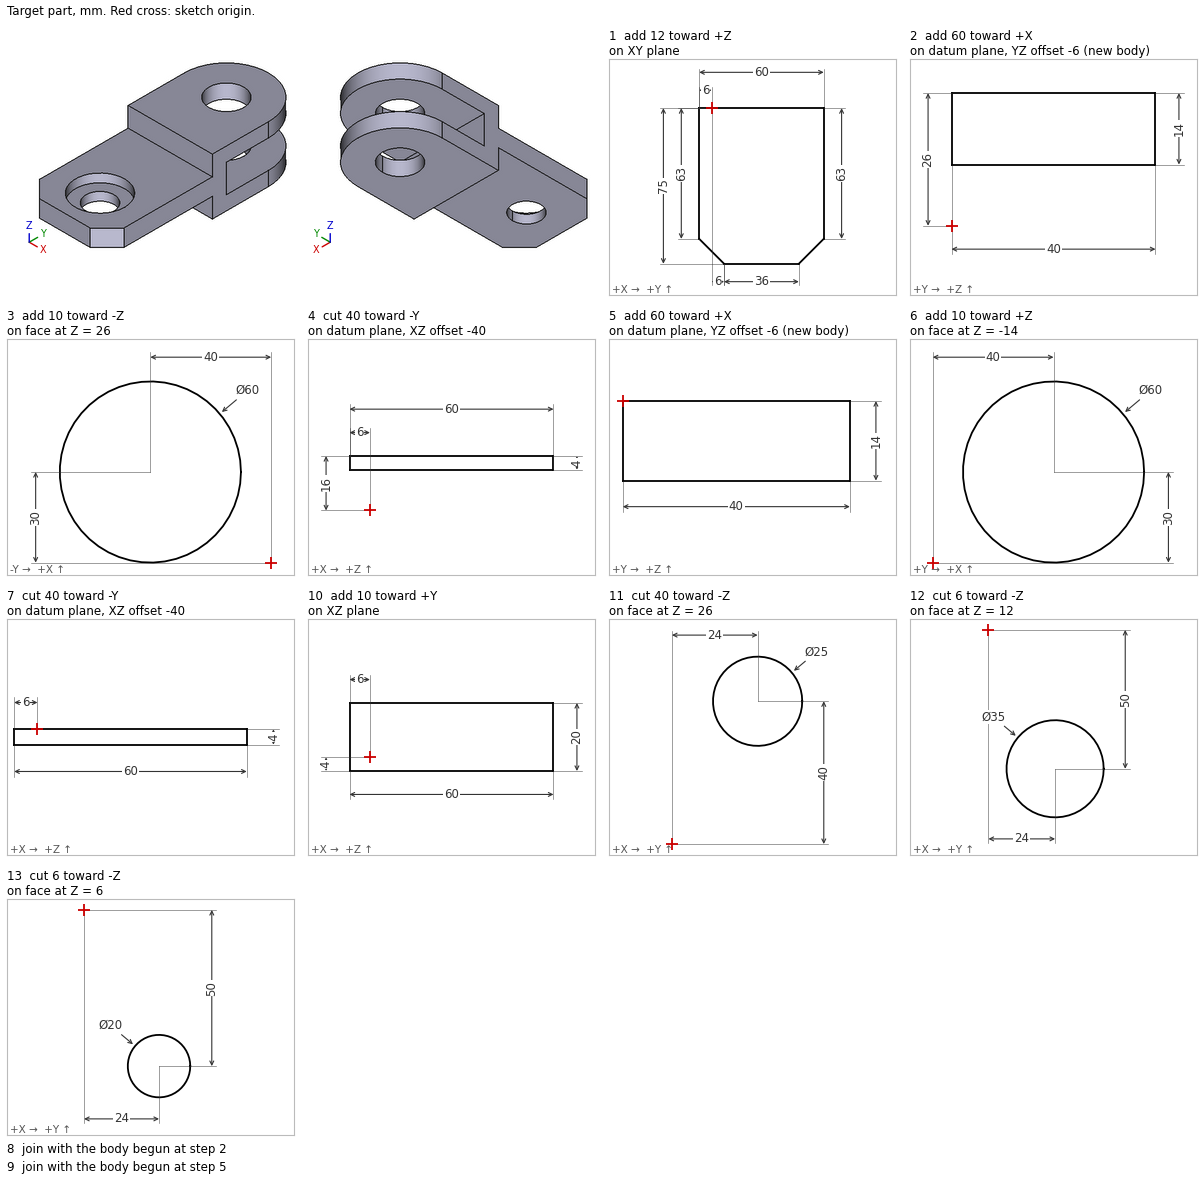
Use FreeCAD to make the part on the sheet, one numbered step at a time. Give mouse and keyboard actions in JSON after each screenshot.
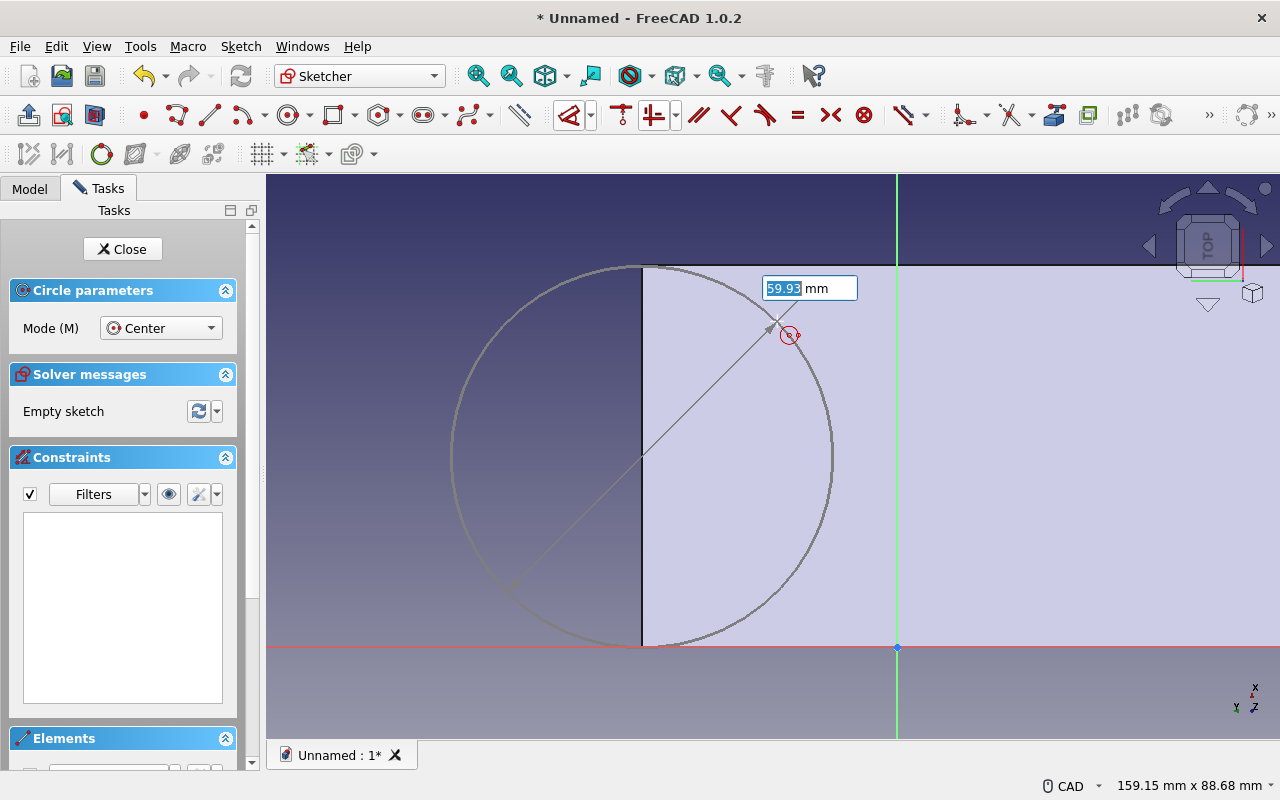
{"action": "type", "text": "60"}
{"action": "key", "text": "Return"}
{"action": "key", "text": "Escape"}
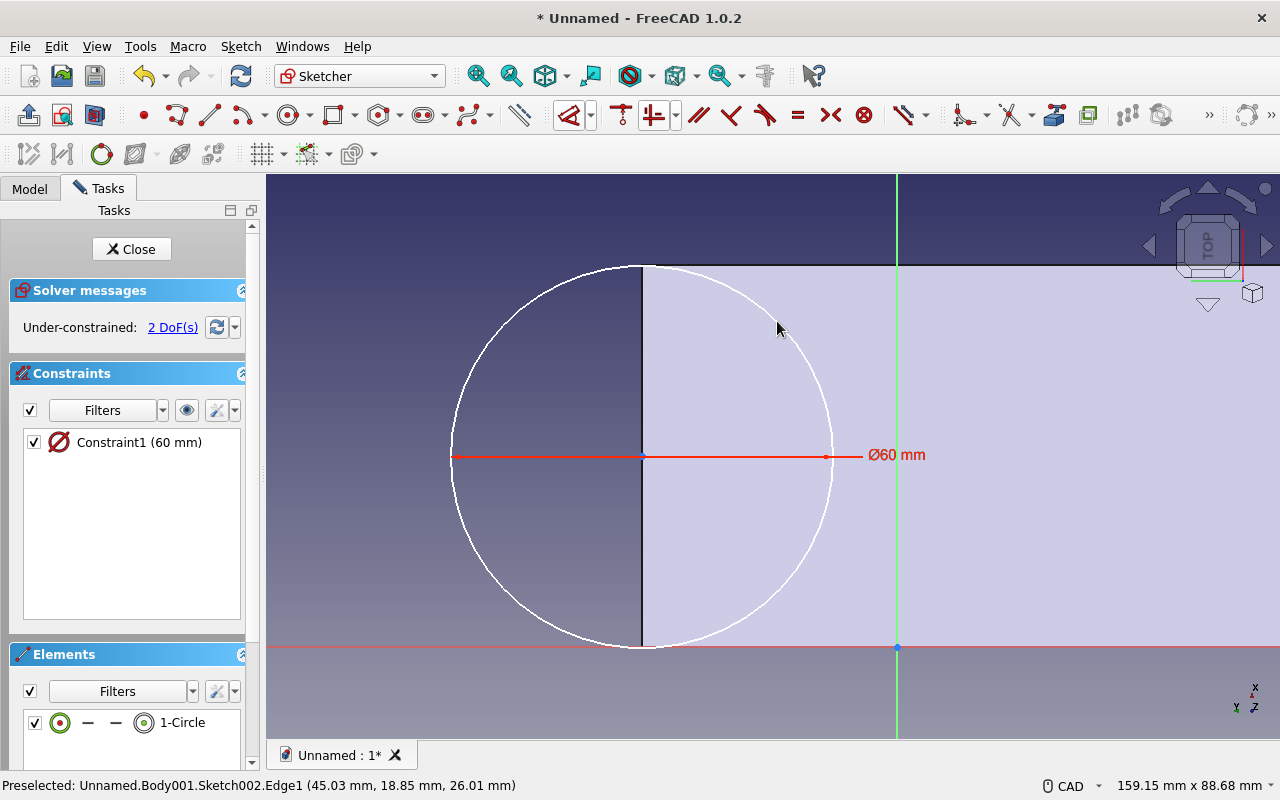
{"action": "left_click", "coordinate": [642, 457]}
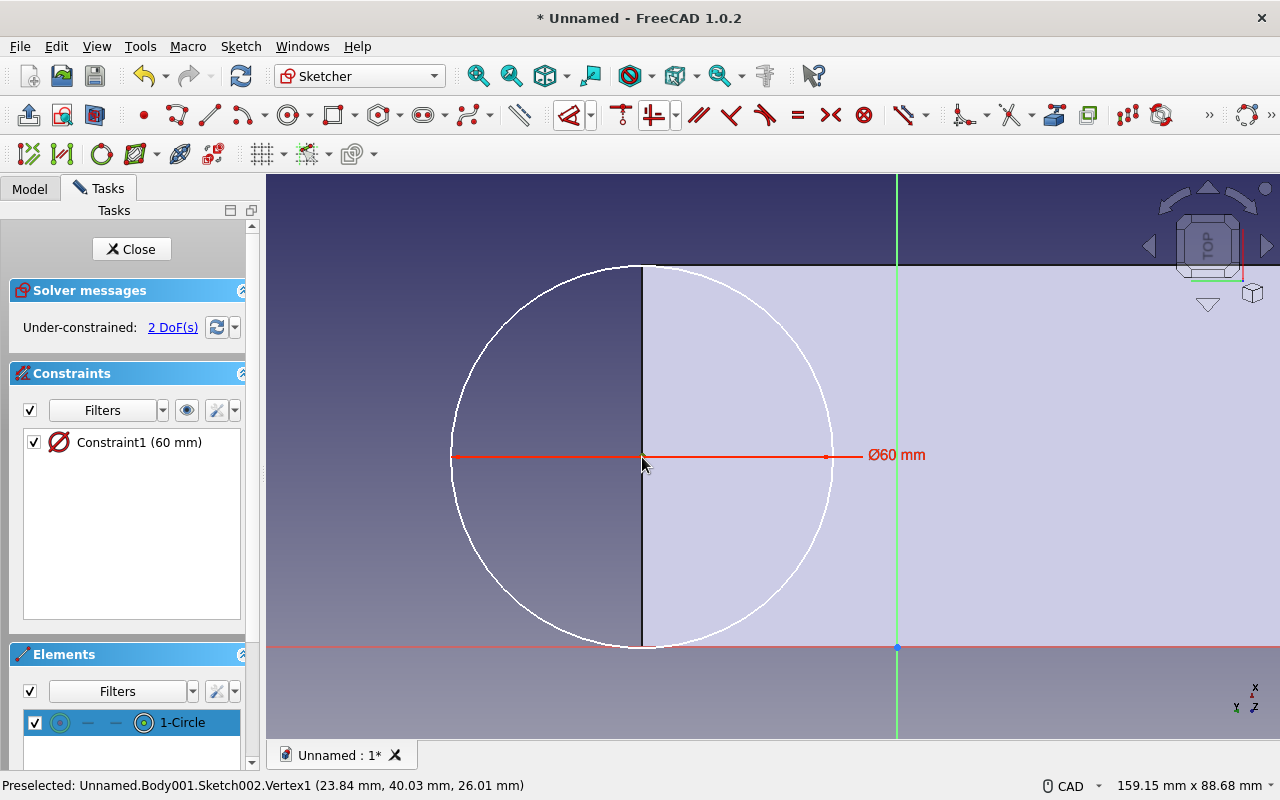
{"action": "left_click", "coordinate": [590, 116]}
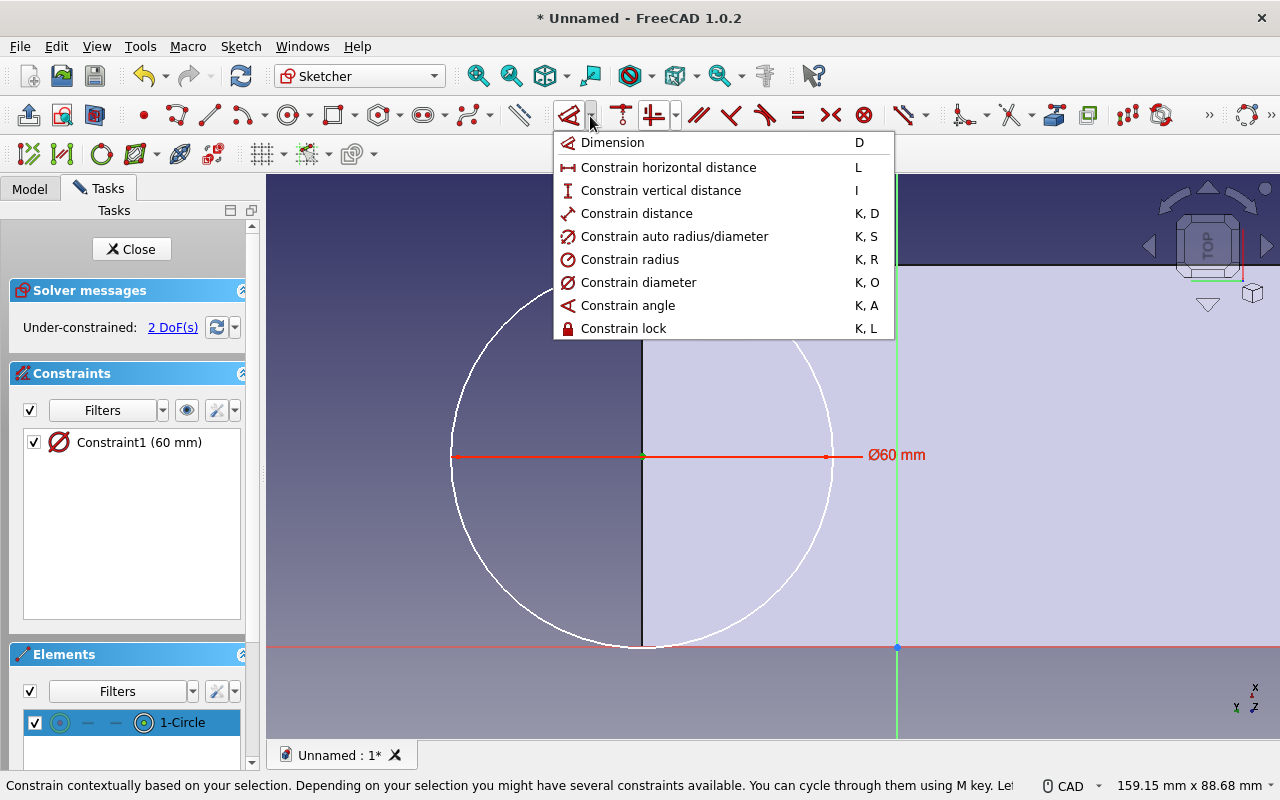
{"action": "left_click", "coordinate": [724, 168]}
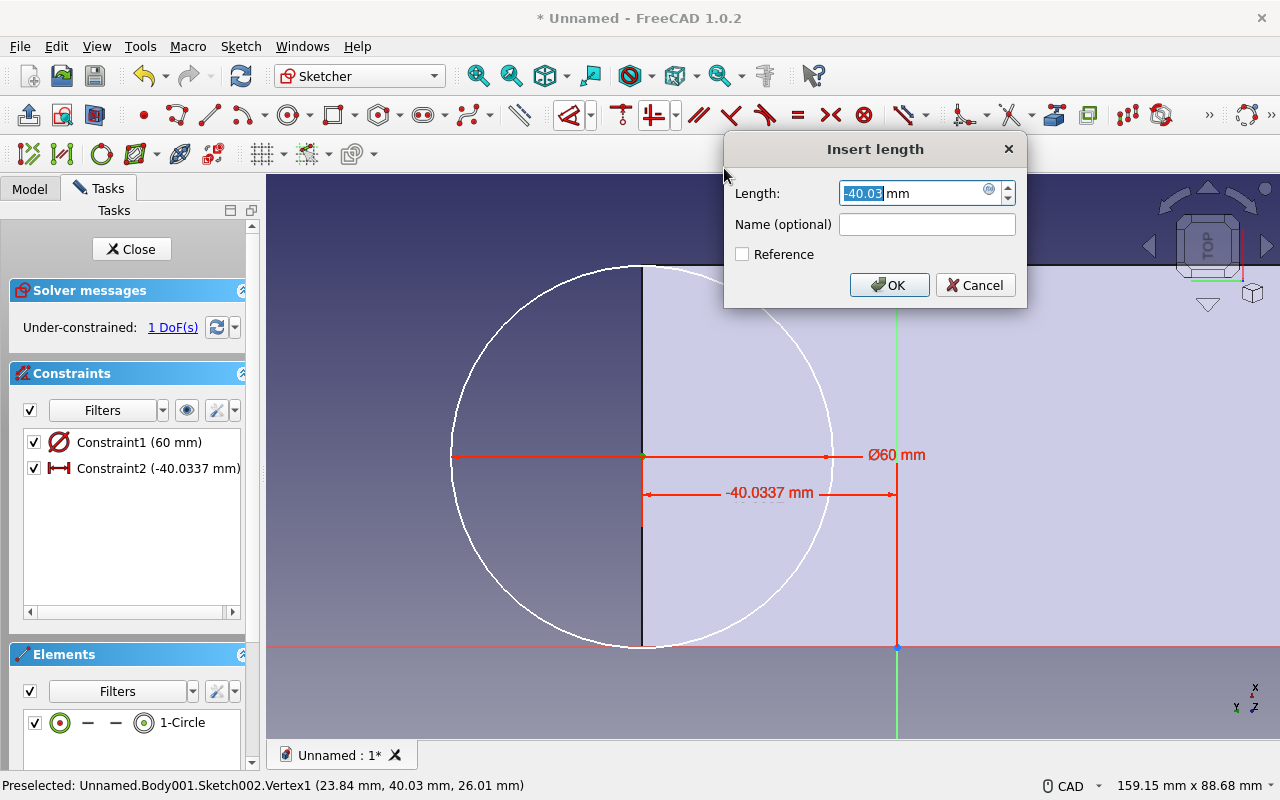
{"action": "type", "text": "-40"}
{"action": "key", "text": "Return"}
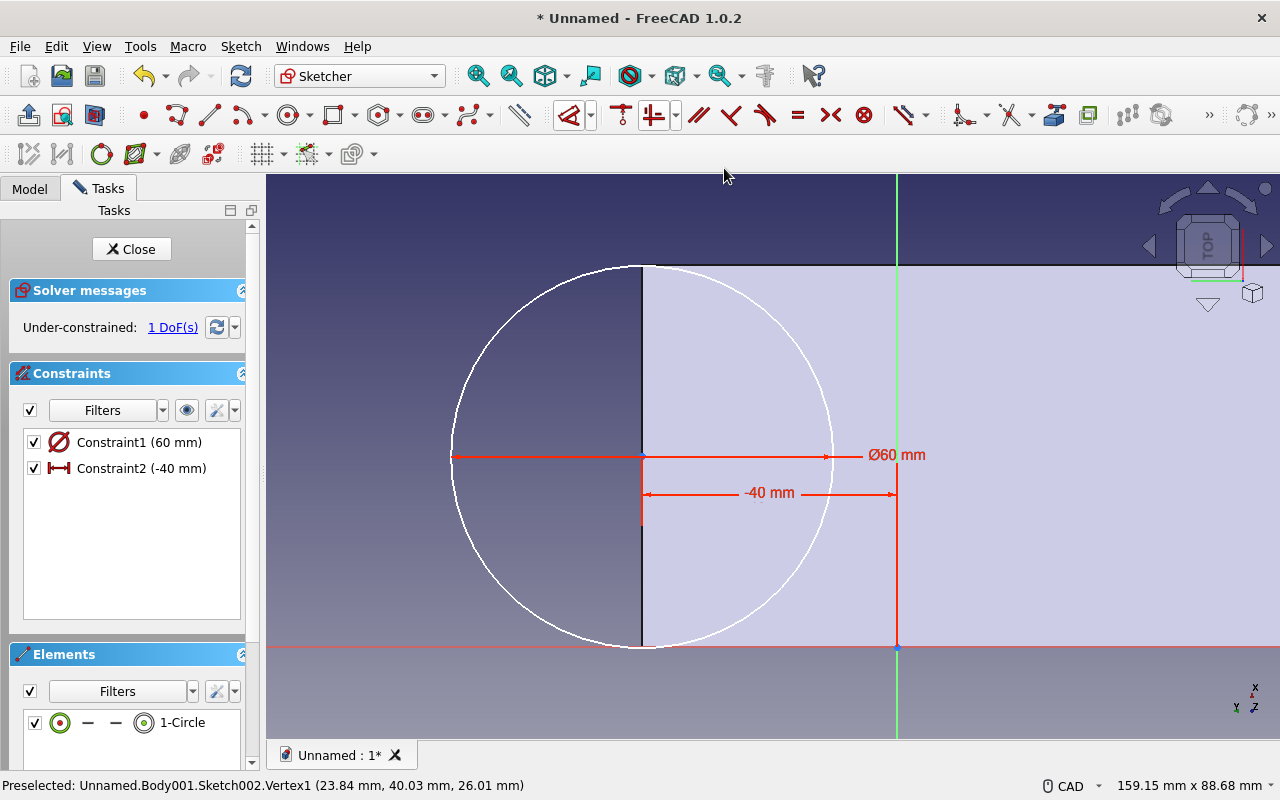
{"action": "left_click", "coordinate": [642, 457]}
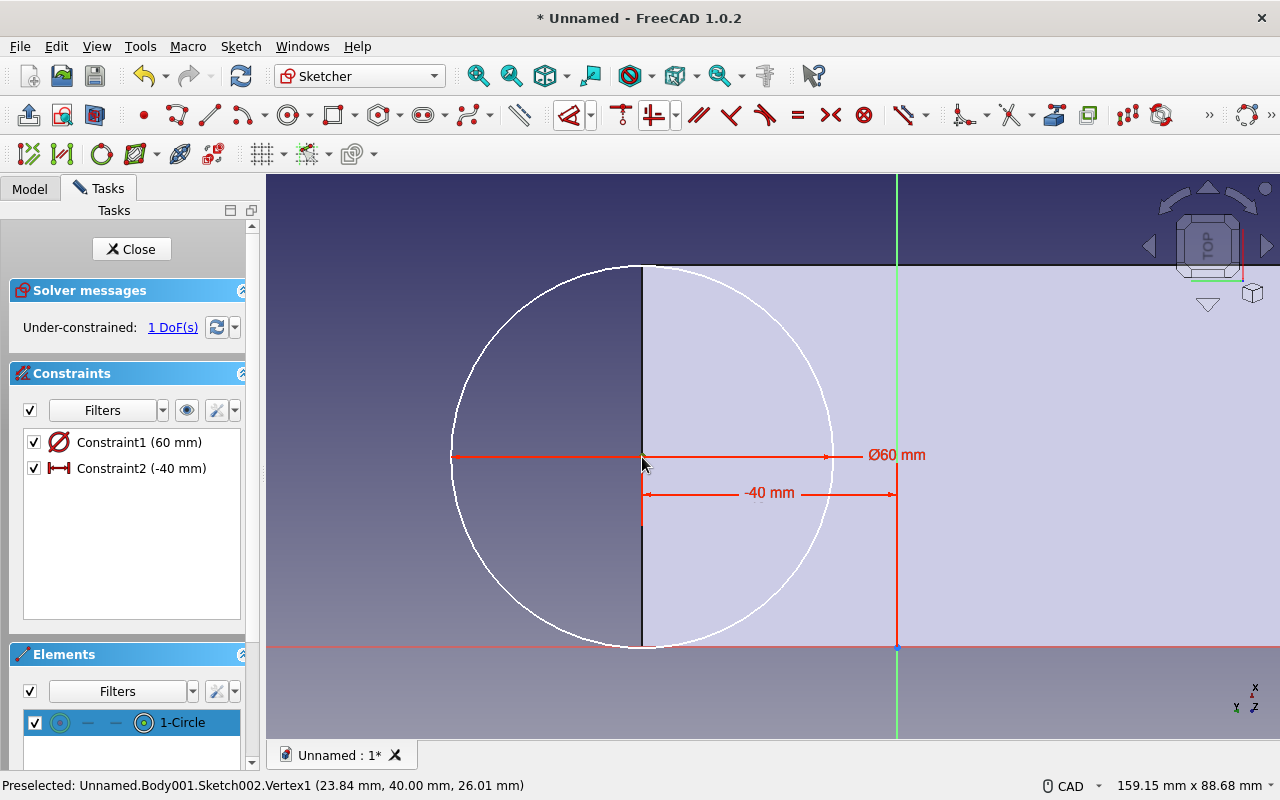
{"action": "left_click", "coordinate": [590, 116]}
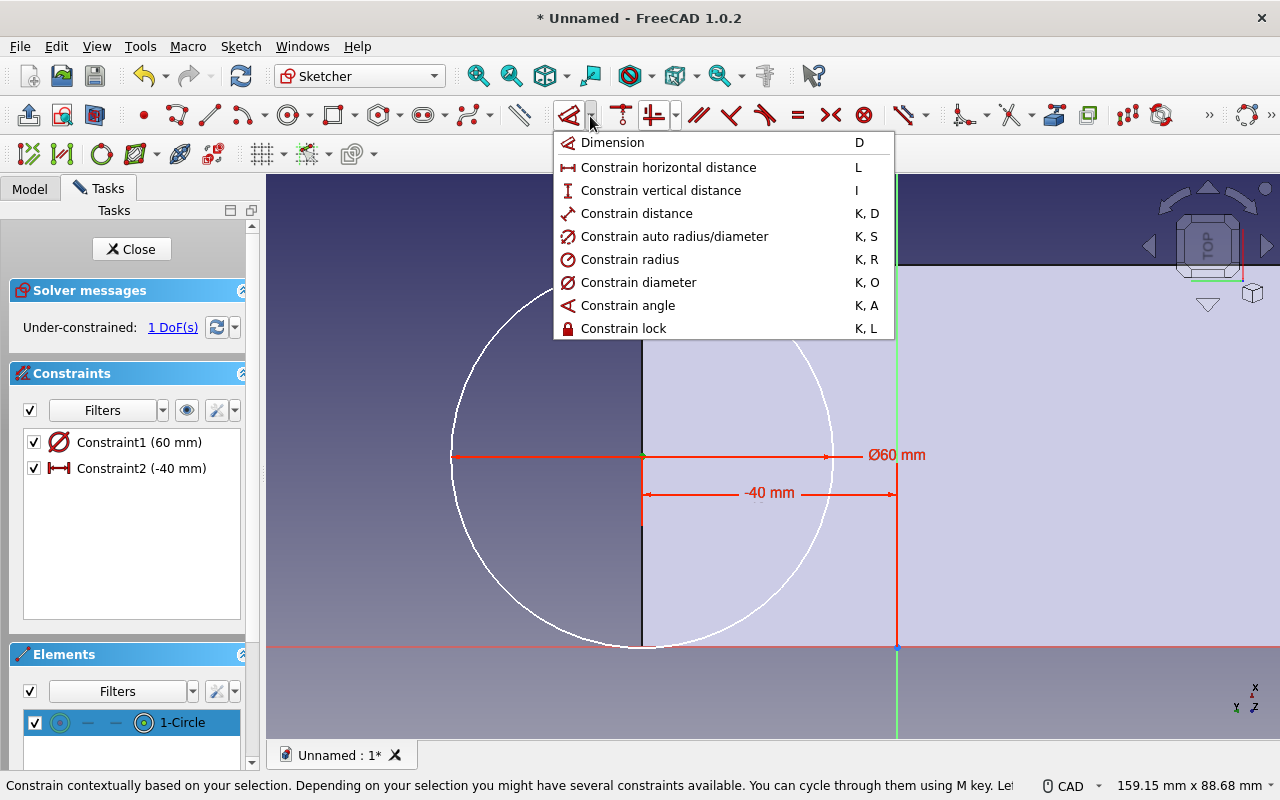
{"action": "left_click", "coordinate": [724, 190]}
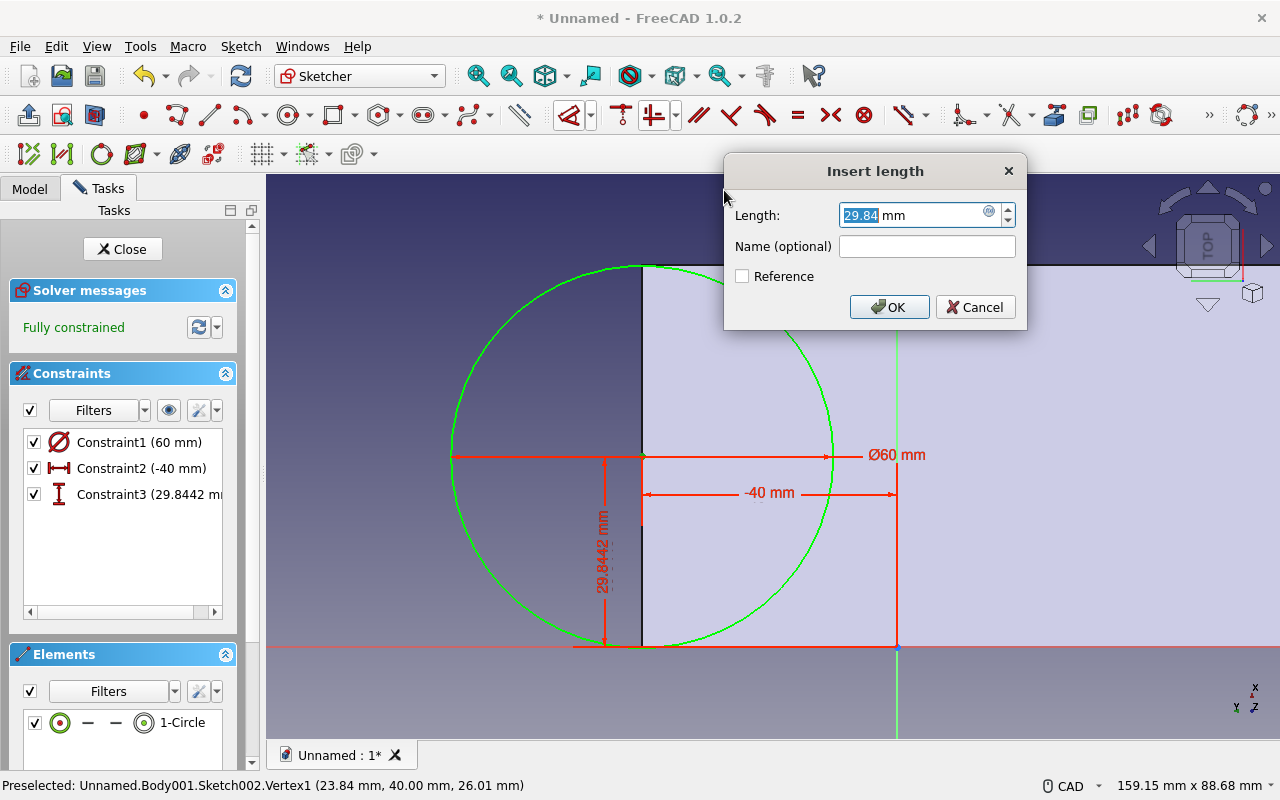
{"action": "type", "text": "30"}
{"action": "key", "text": "Return"}